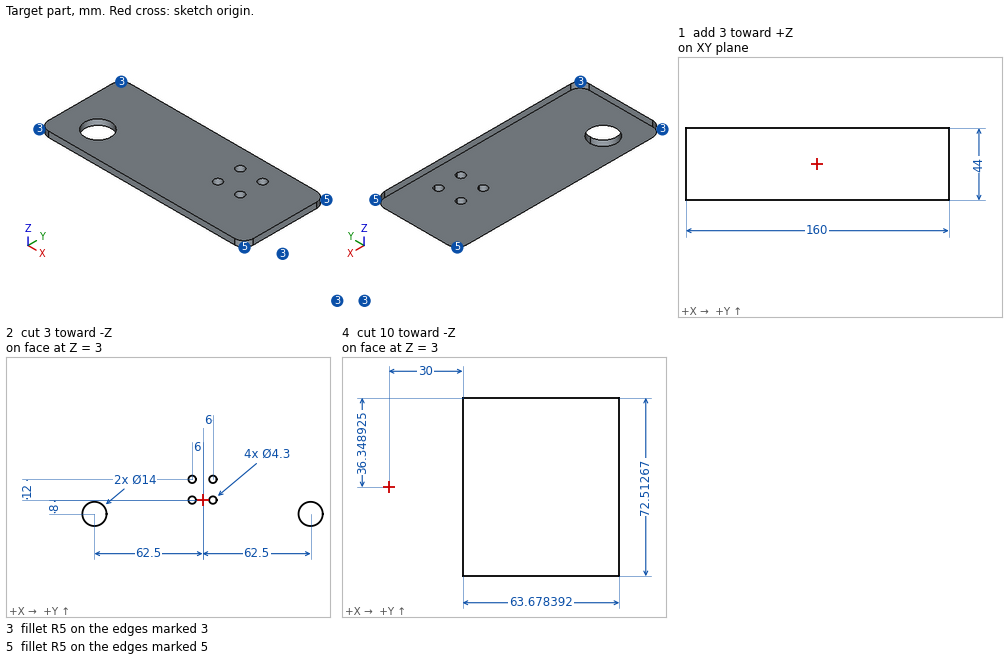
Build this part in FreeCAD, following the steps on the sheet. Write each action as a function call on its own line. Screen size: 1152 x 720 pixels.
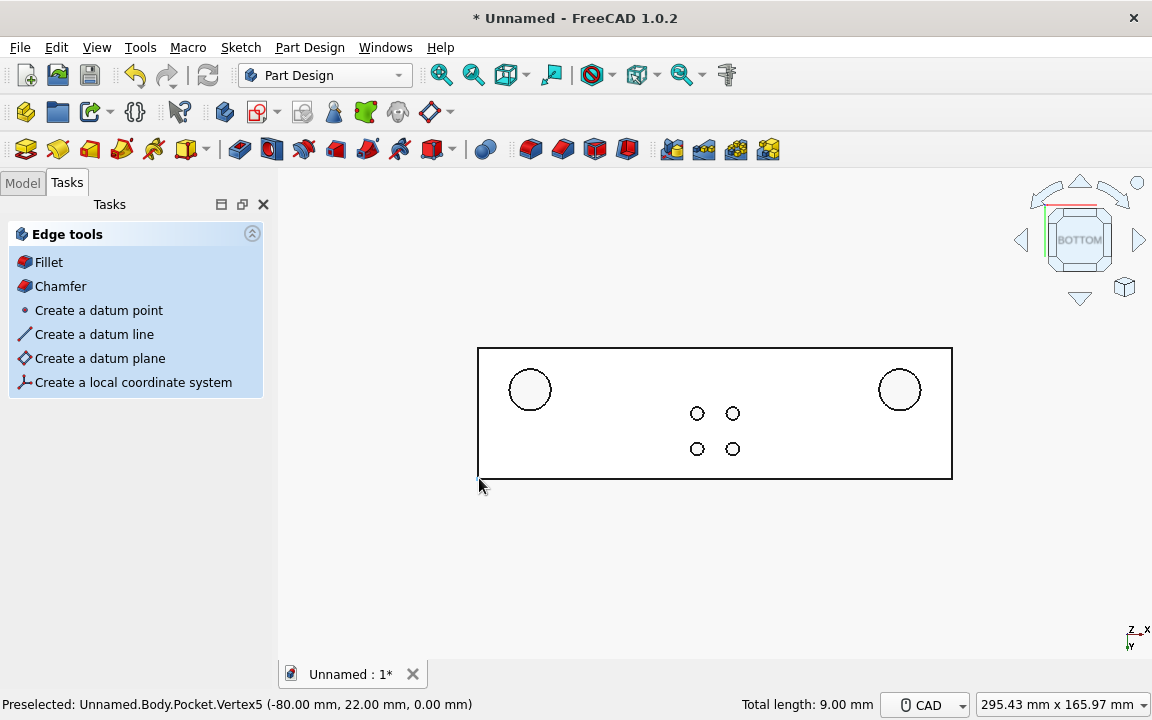
key(4)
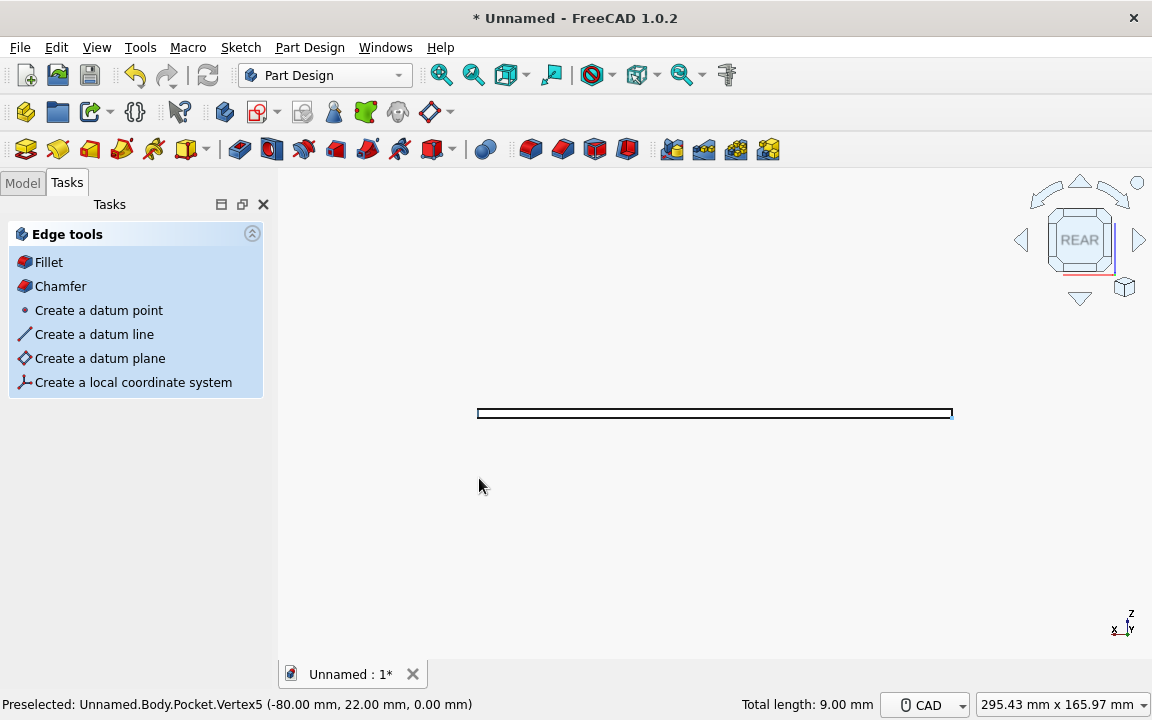
scroll(952, 413, up, 8)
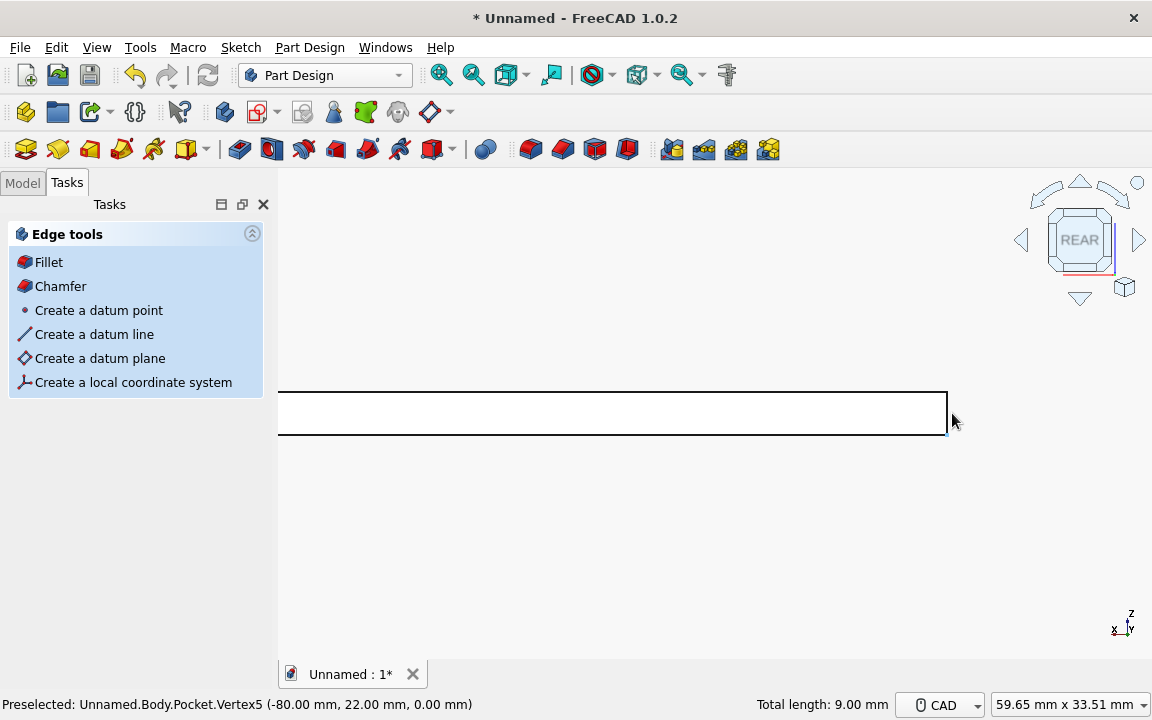
click(947, 413, ctrl)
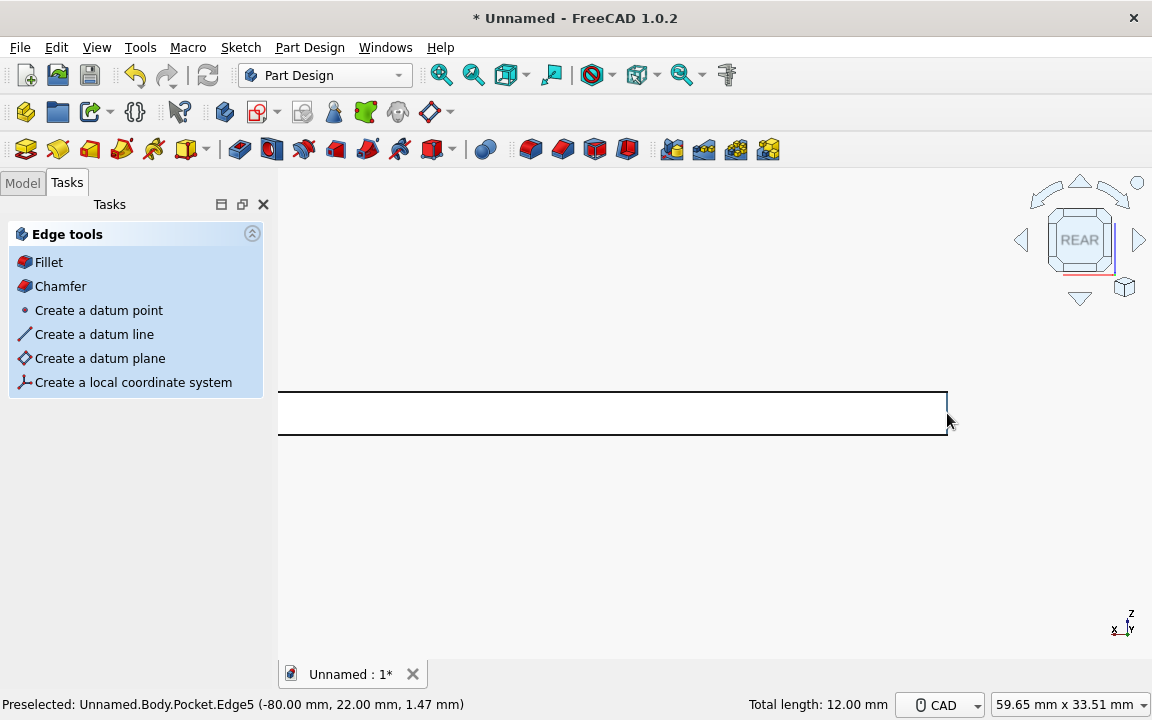
click(532, 150)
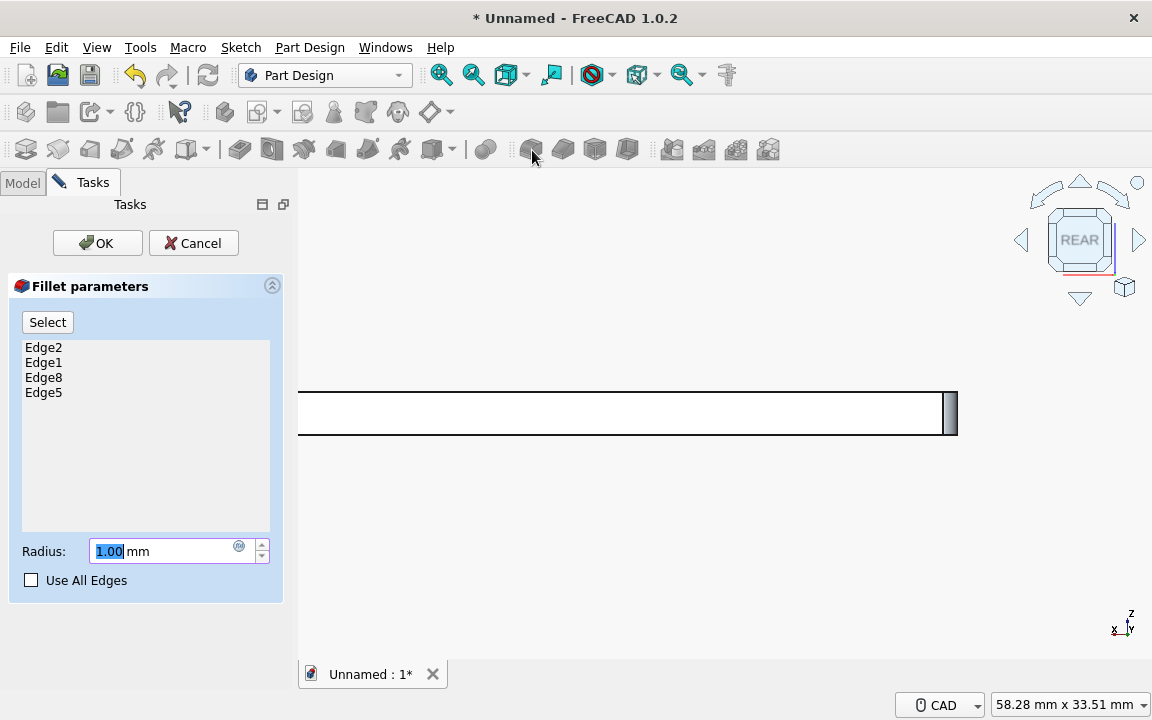
text(5)
key(Tab)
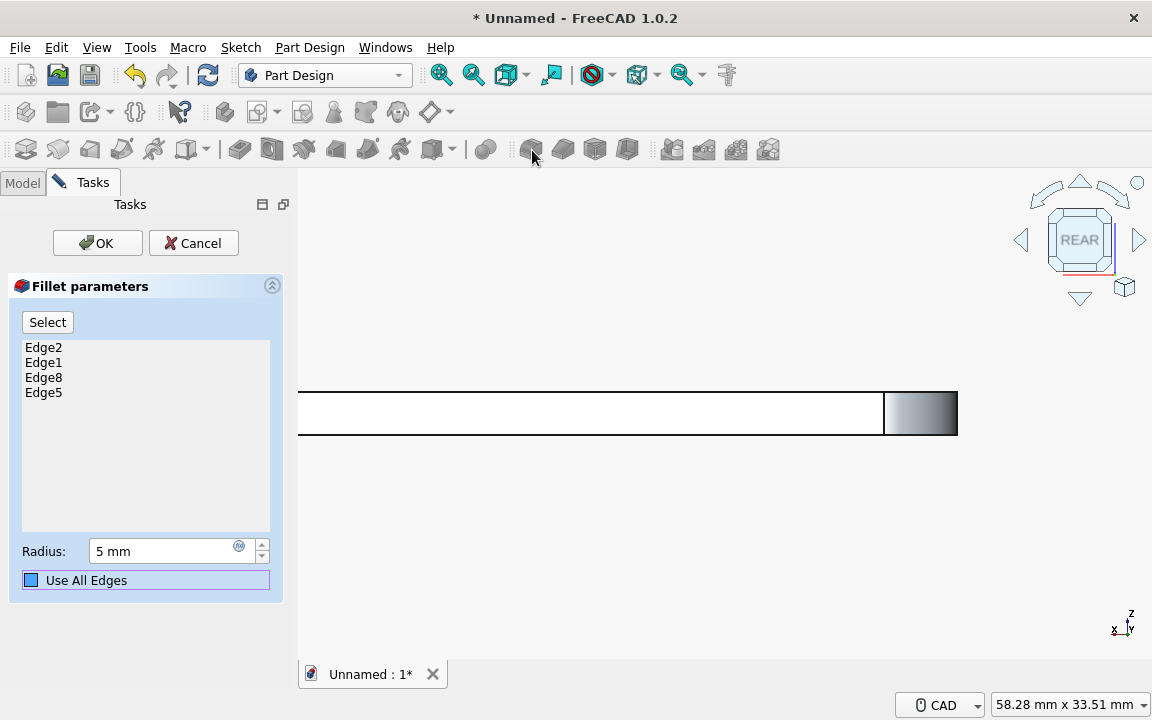
click(98, 243)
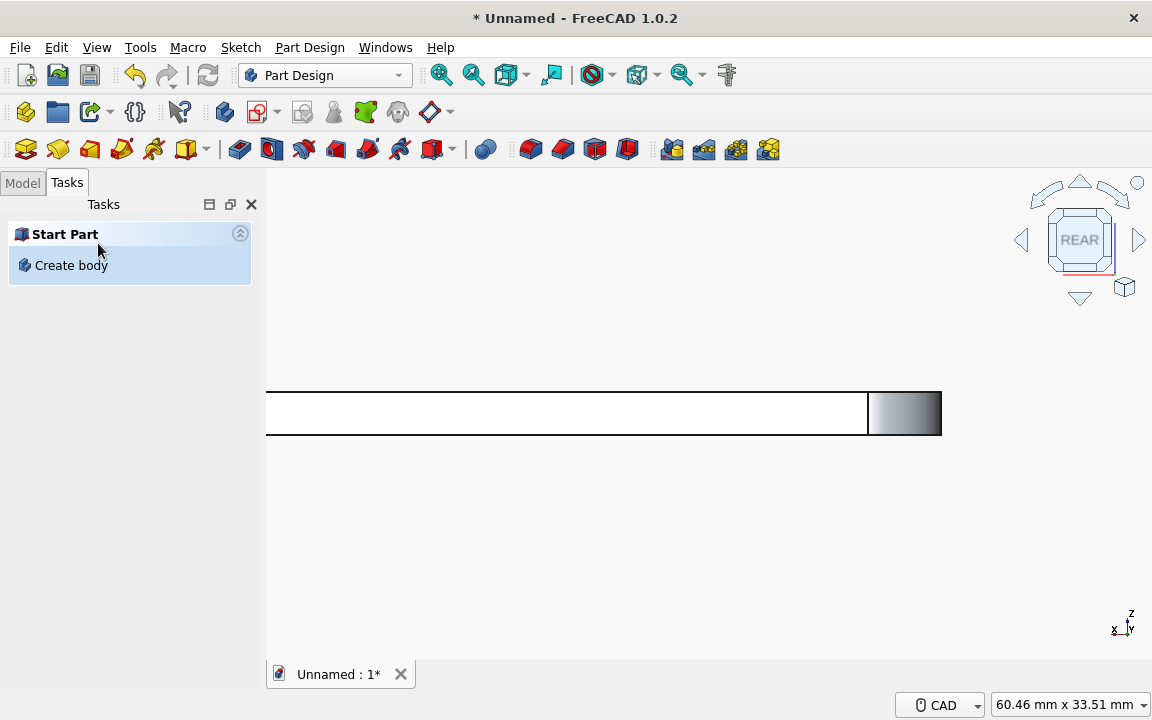
key(v)
key(f)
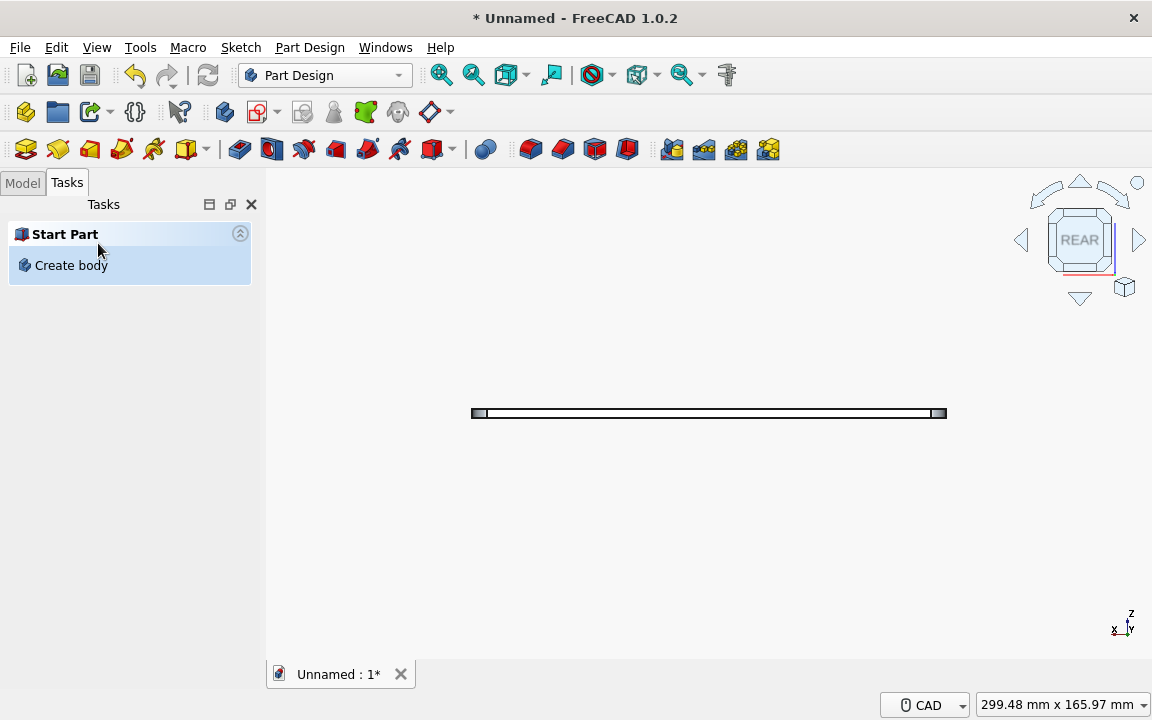
key(0)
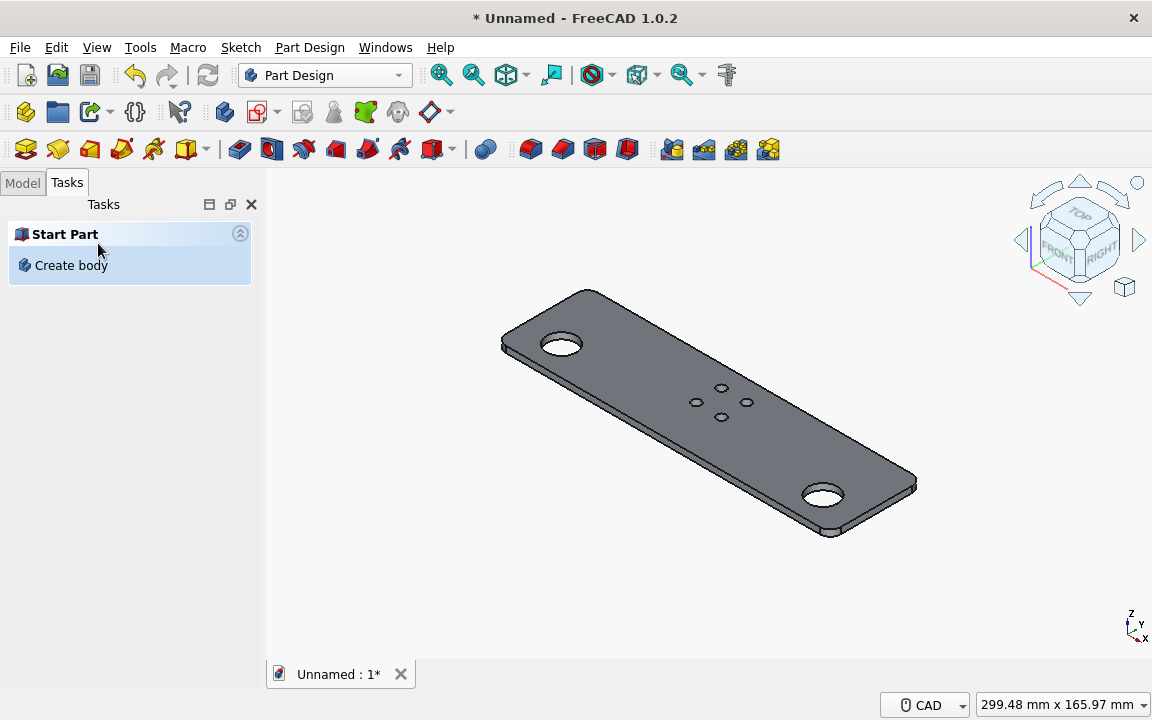
click(744, 444)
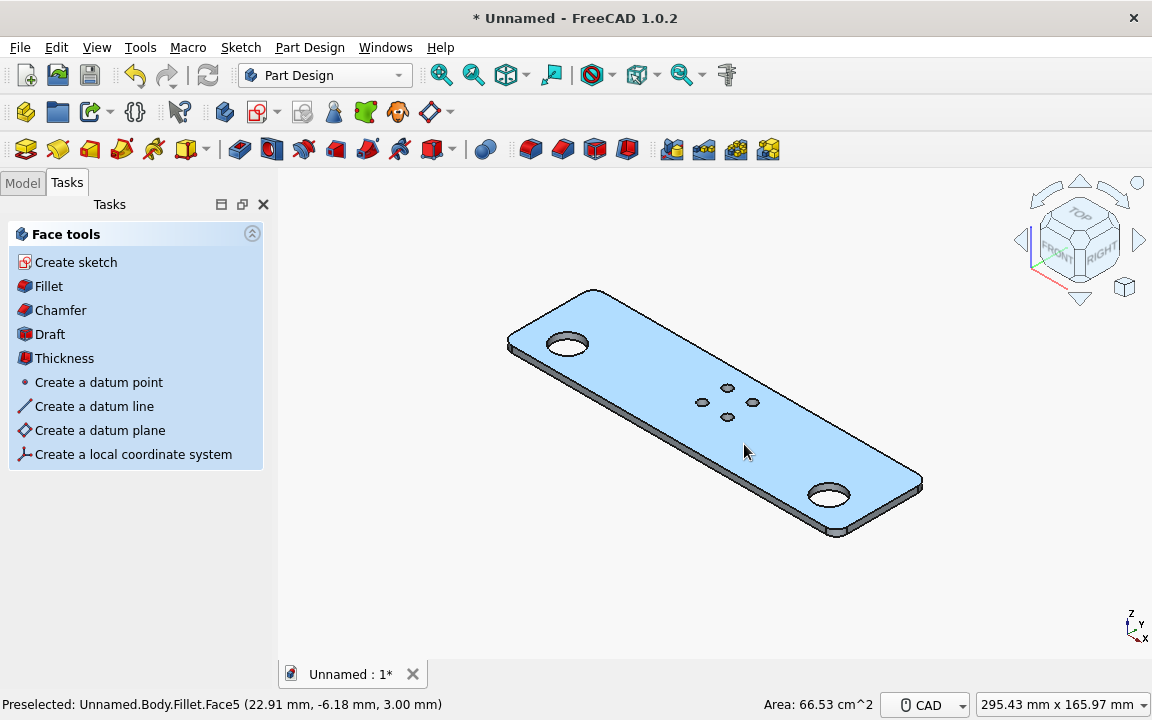
click(258, 112)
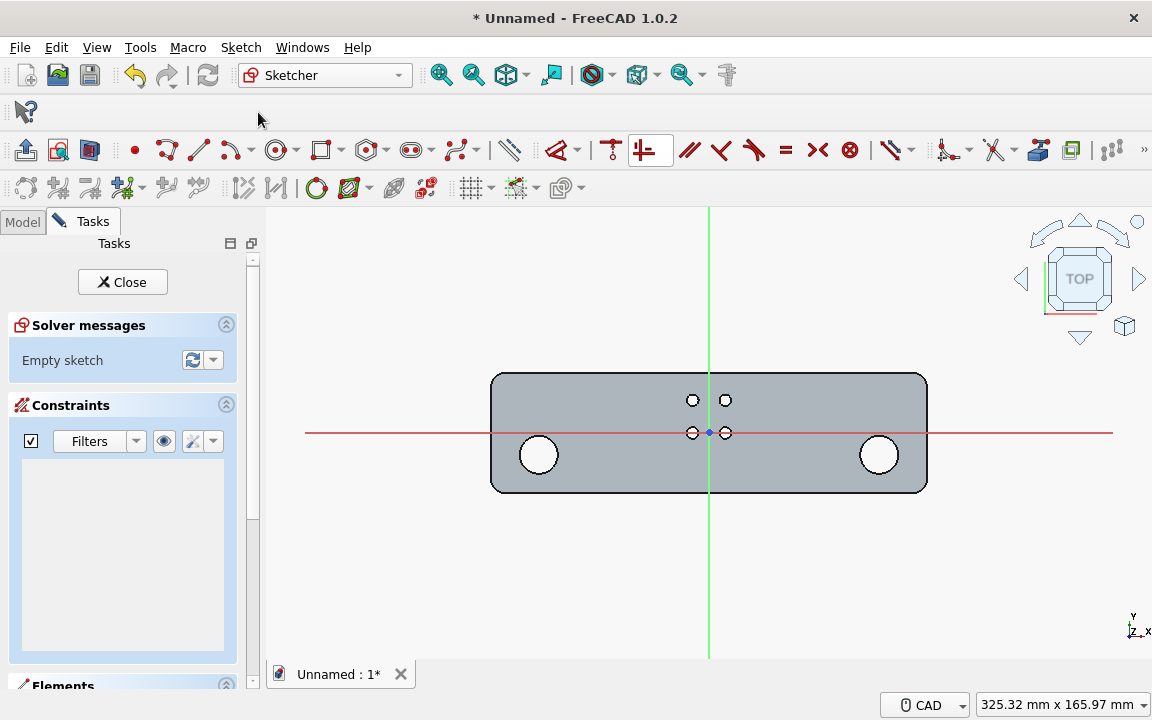
scroll(987, 432, up, 2)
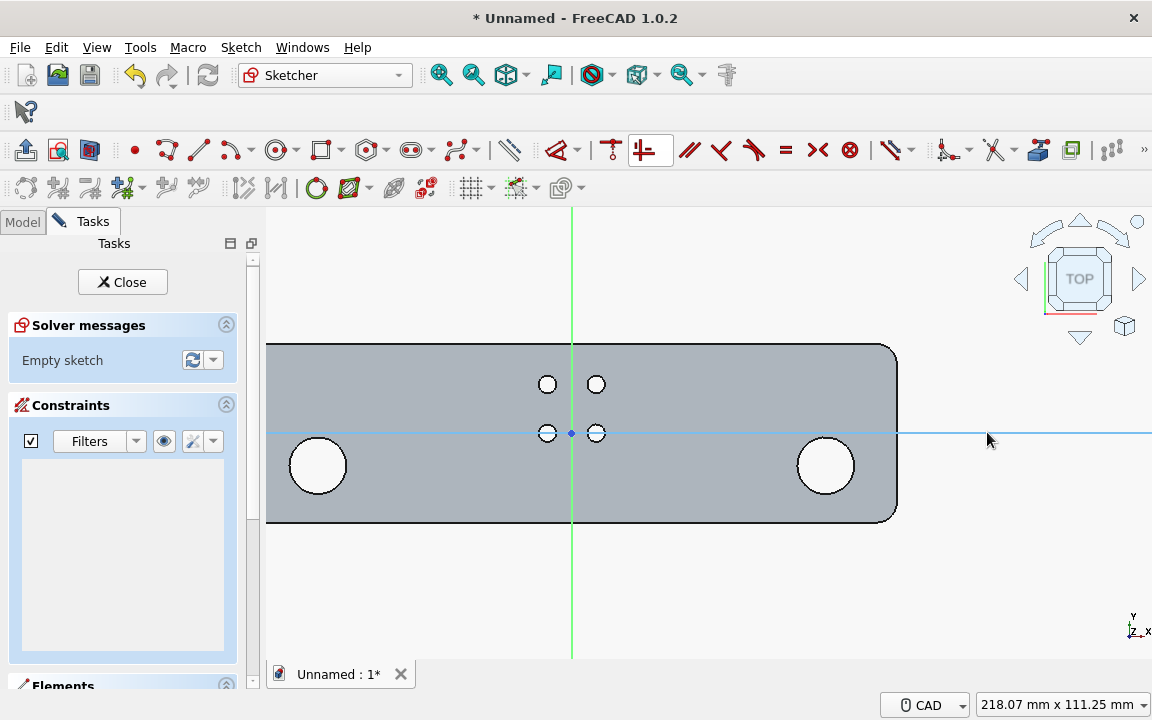
key(g)
key(r)